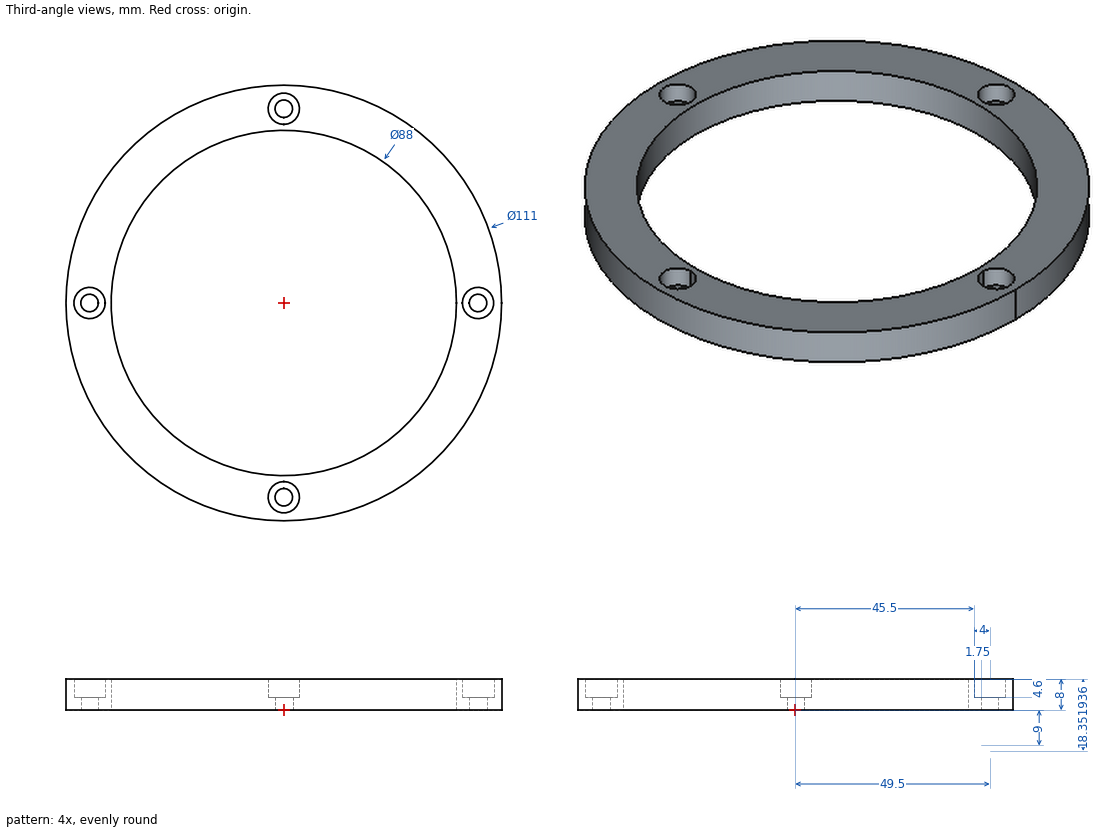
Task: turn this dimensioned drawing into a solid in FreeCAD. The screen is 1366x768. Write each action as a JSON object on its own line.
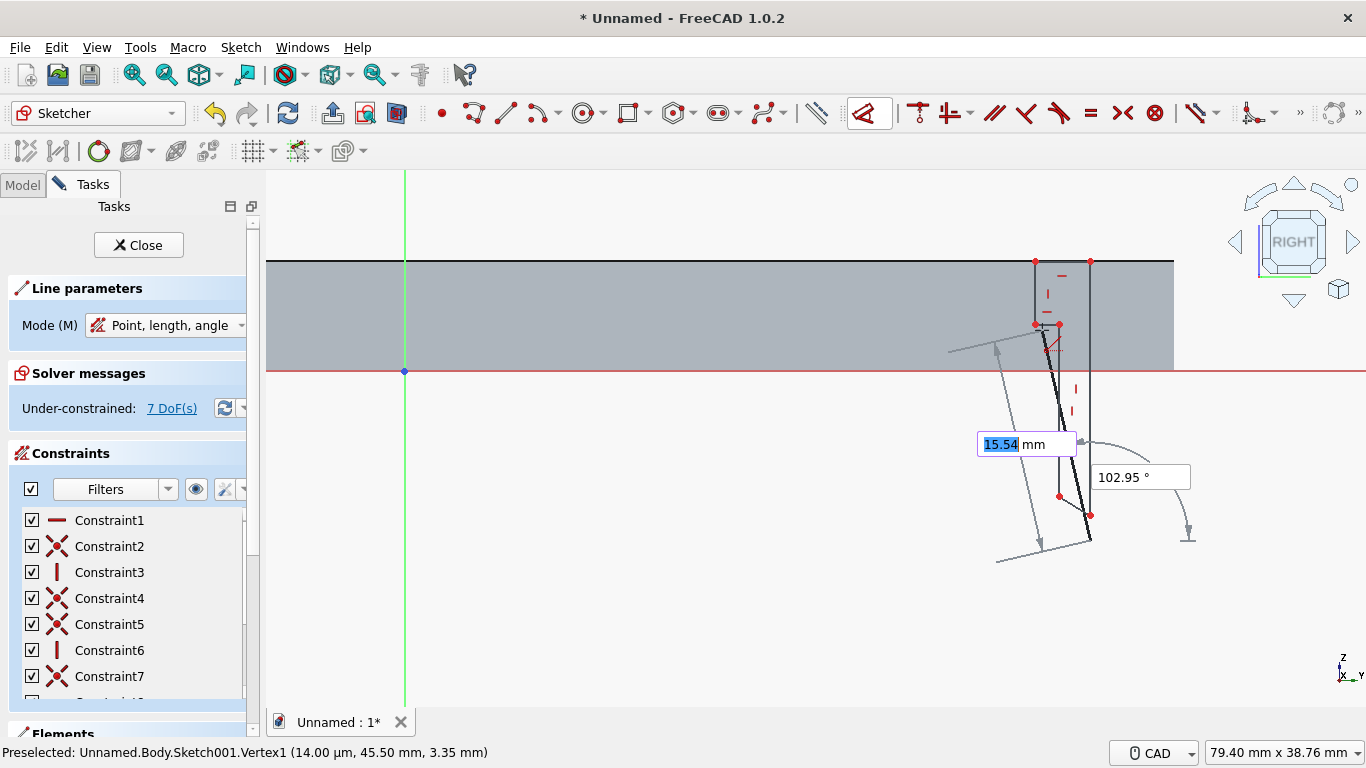
{"action": "left_click", "coordinate": [1090, 617]}
{"action": "key", "text": "Escape"}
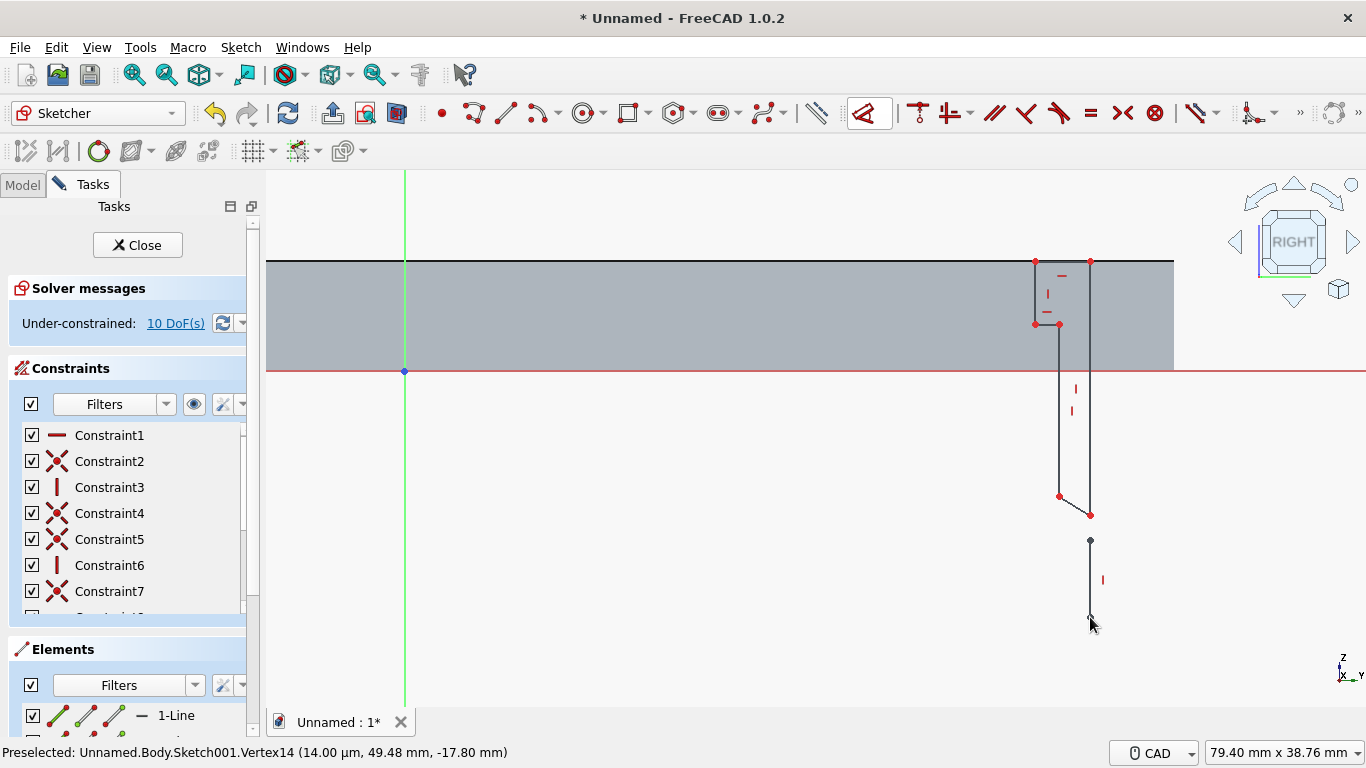
{"action": "left_click", "coordinate": [1090, 564]}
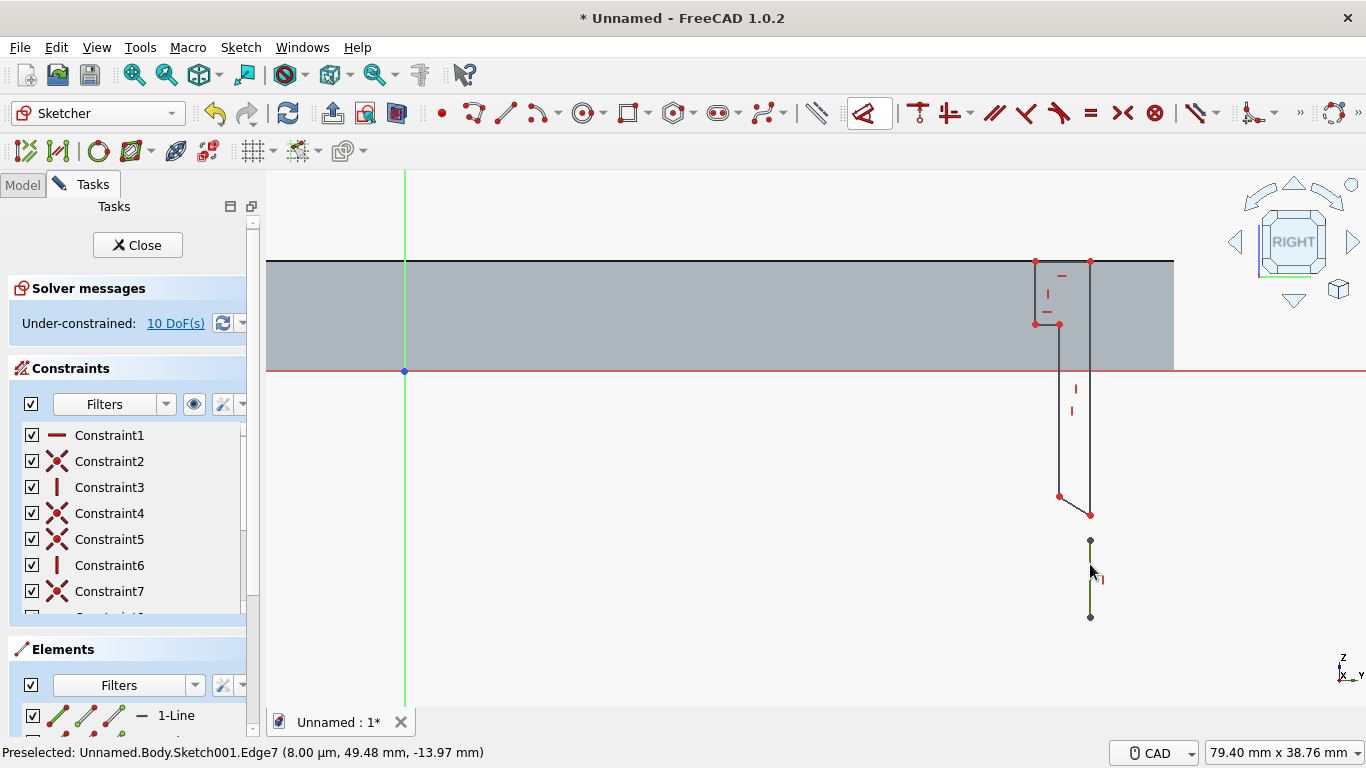
{"action": "left_click", "coordinate": [818, 114]}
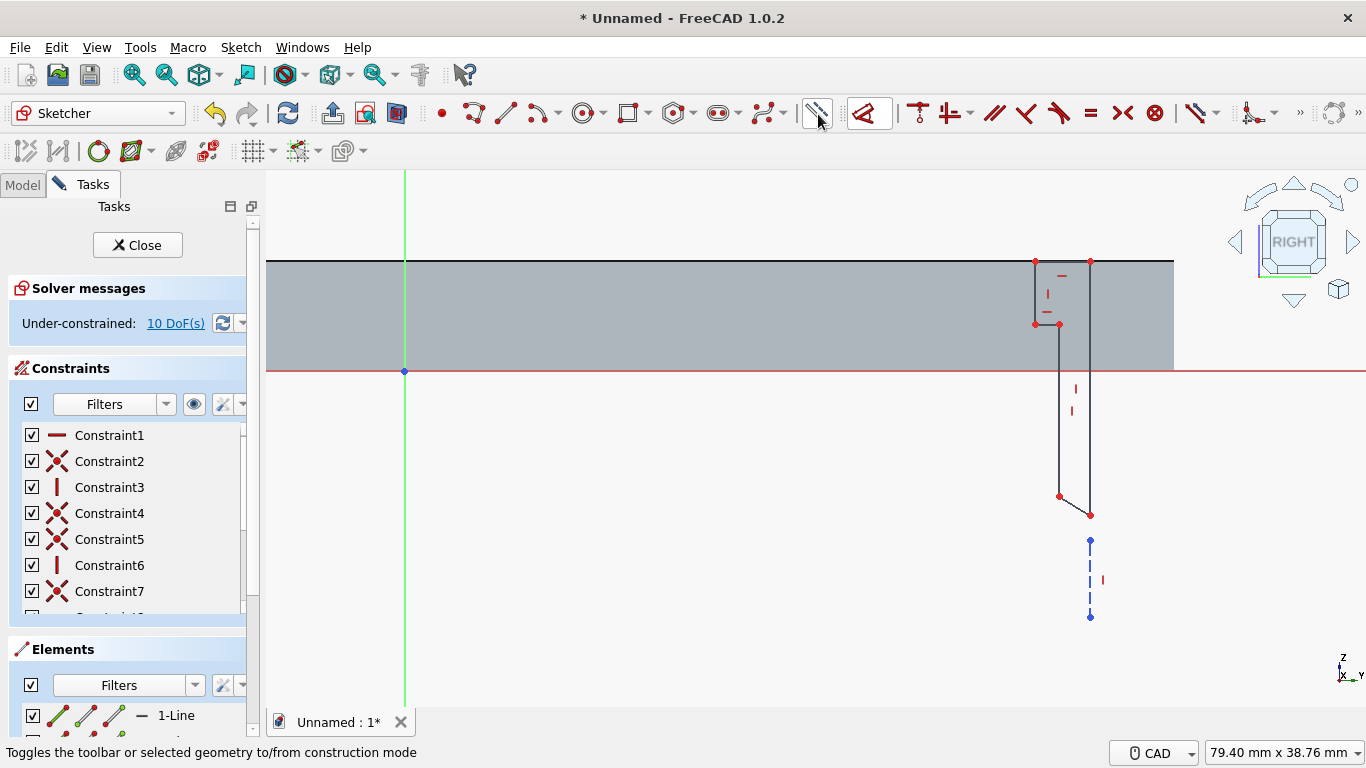
{"action": "left_click", "coordinate": [864, 114]}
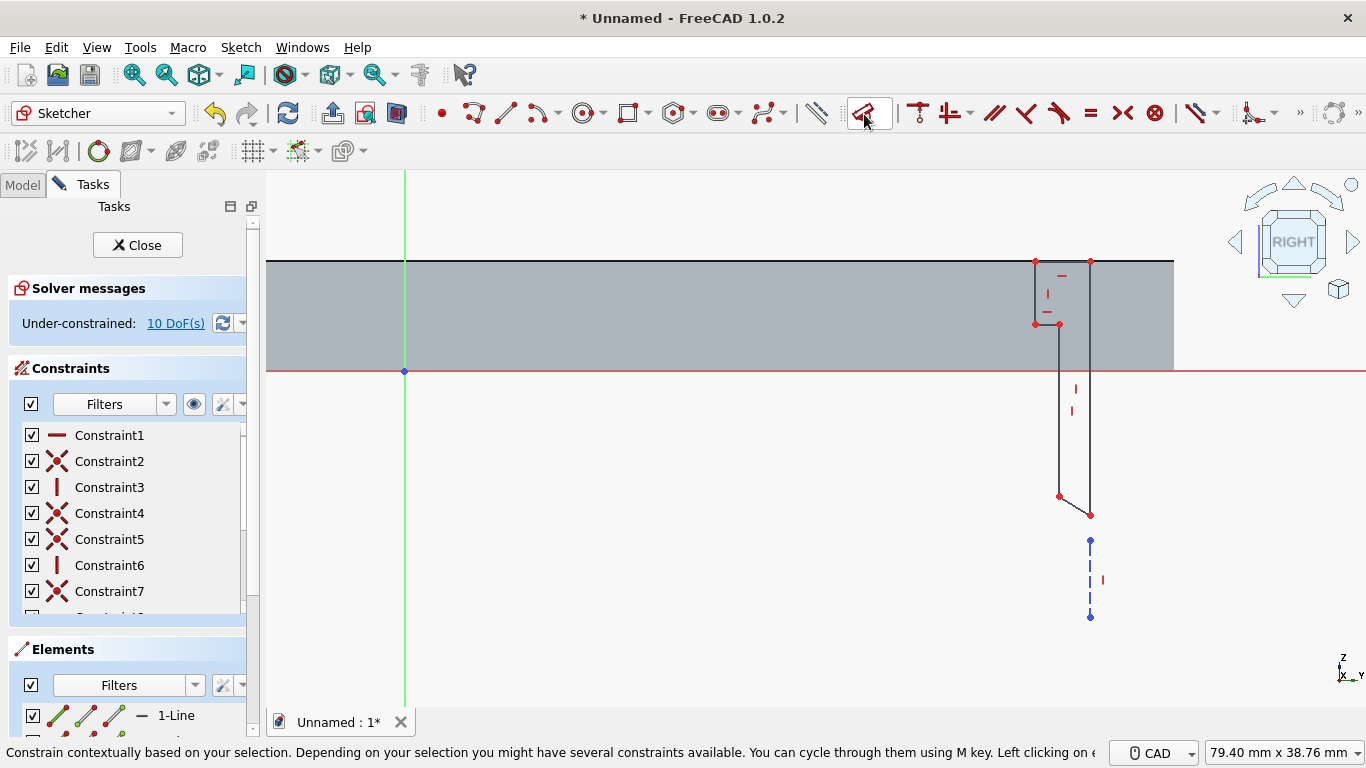
{"action": "left_click", "coordinate": [1074, 262]}
{"action": "left_click", "coordinate": [1063, 228]}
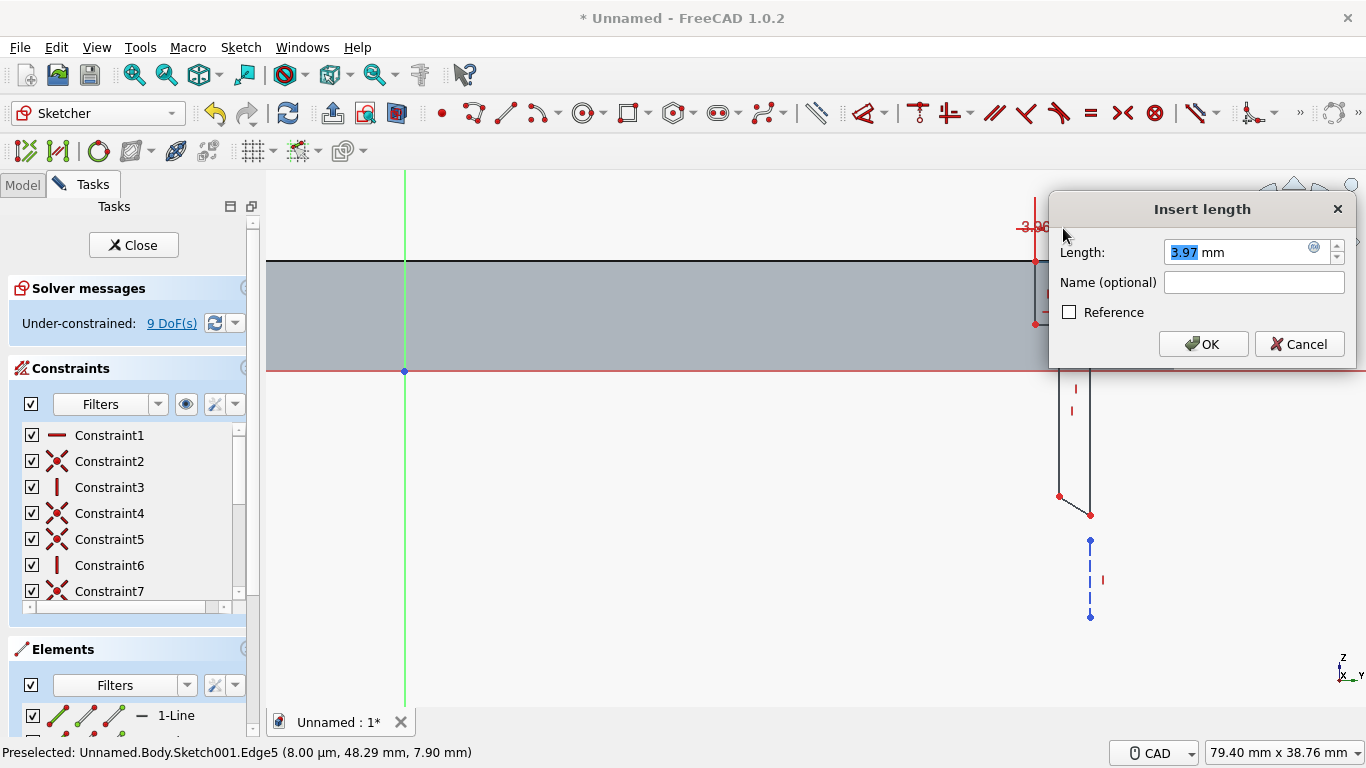
{"action": "type", "text": "4"}
{"action": "key", "text": "Return"}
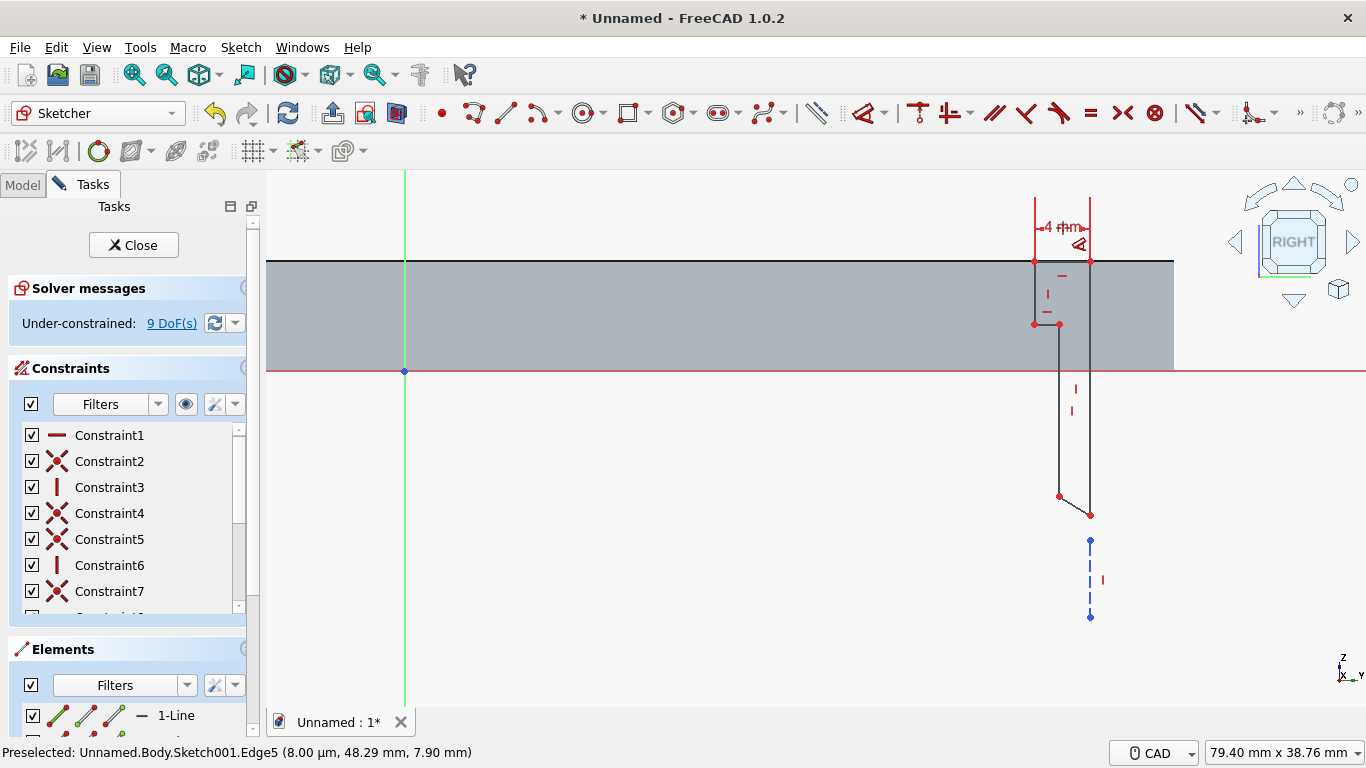
{"action": "left_click", "coordinate": [1059, 497]}
{"action": "left_click", "coordinate": [371, 434]}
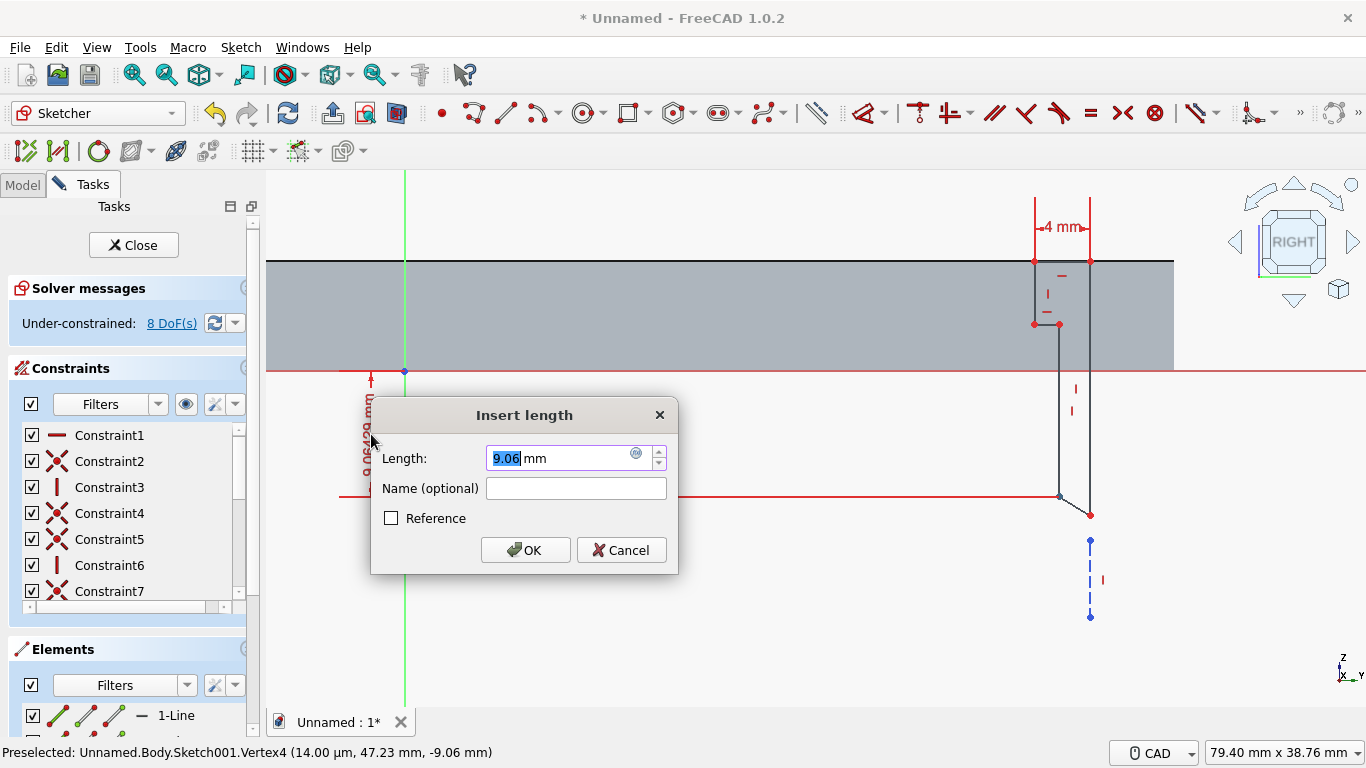
{"action": "type", "text": "9"}
{"action": "key", "text": "Return"}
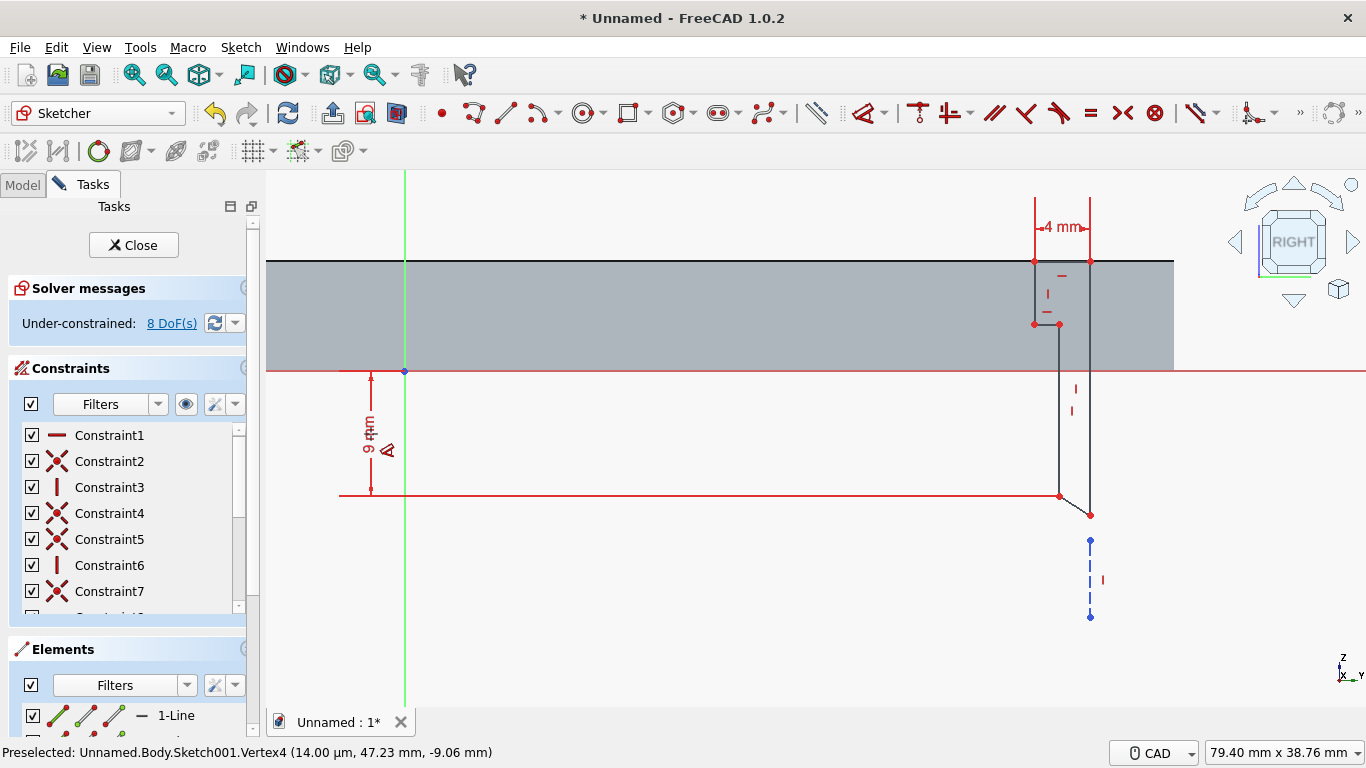
{"action": "left_click", "coordinate": [1090, 262]}
{"action": "left_click", "coordinate": [371, 317]}